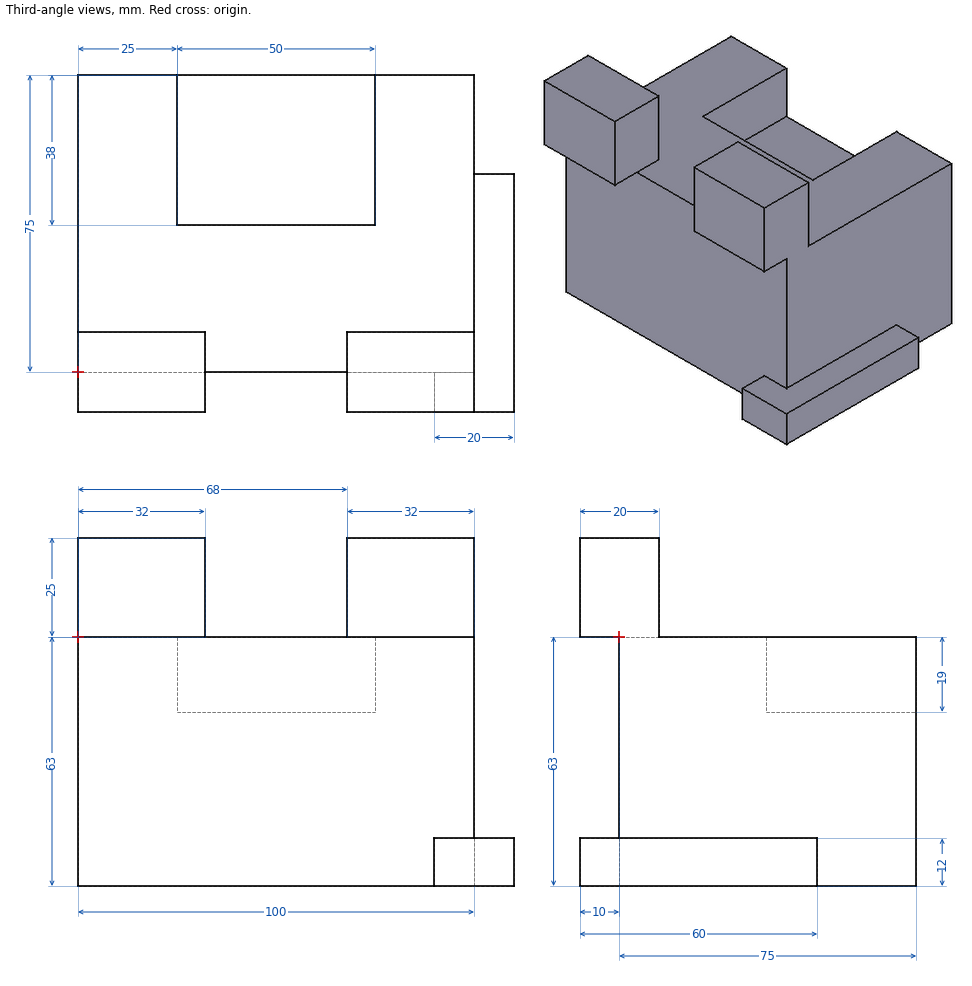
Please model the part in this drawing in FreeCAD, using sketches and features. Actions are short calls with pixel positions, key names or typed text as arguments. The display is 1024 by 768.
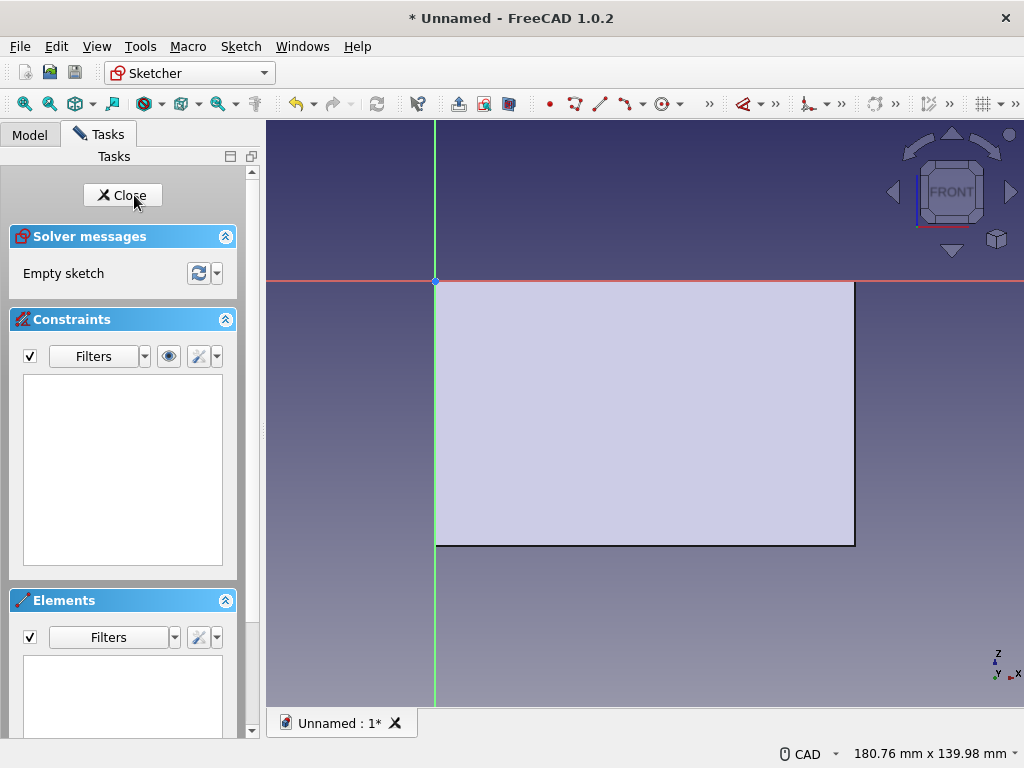
scroll(294, 679, down, 1)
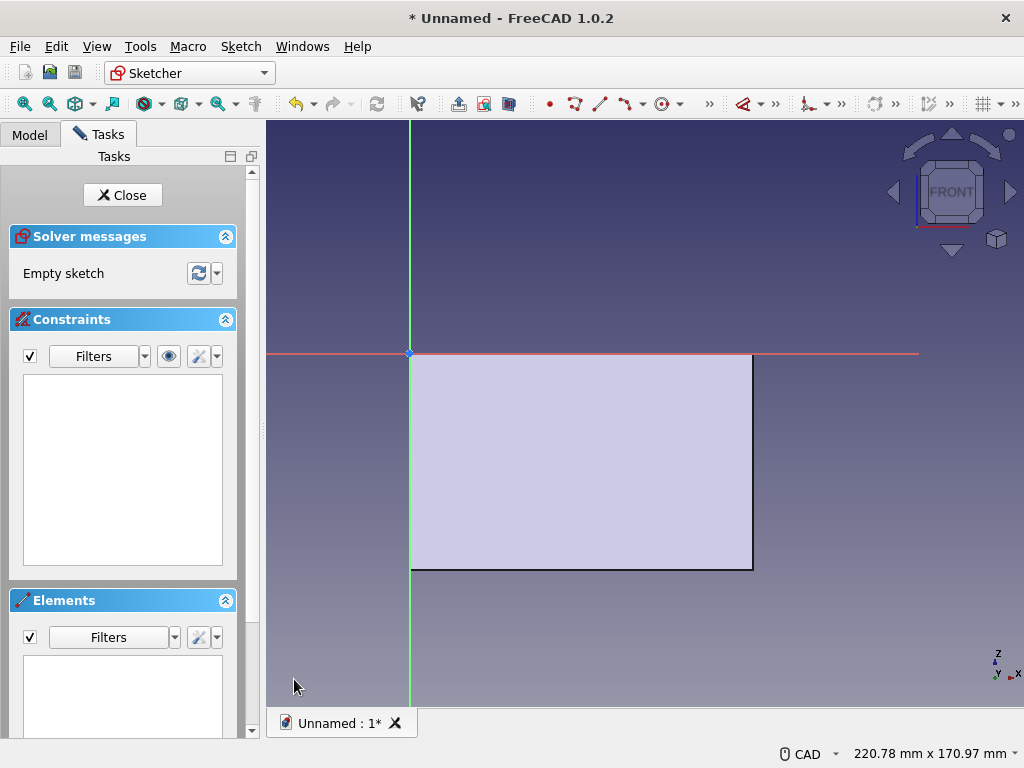
key(g)
key(r)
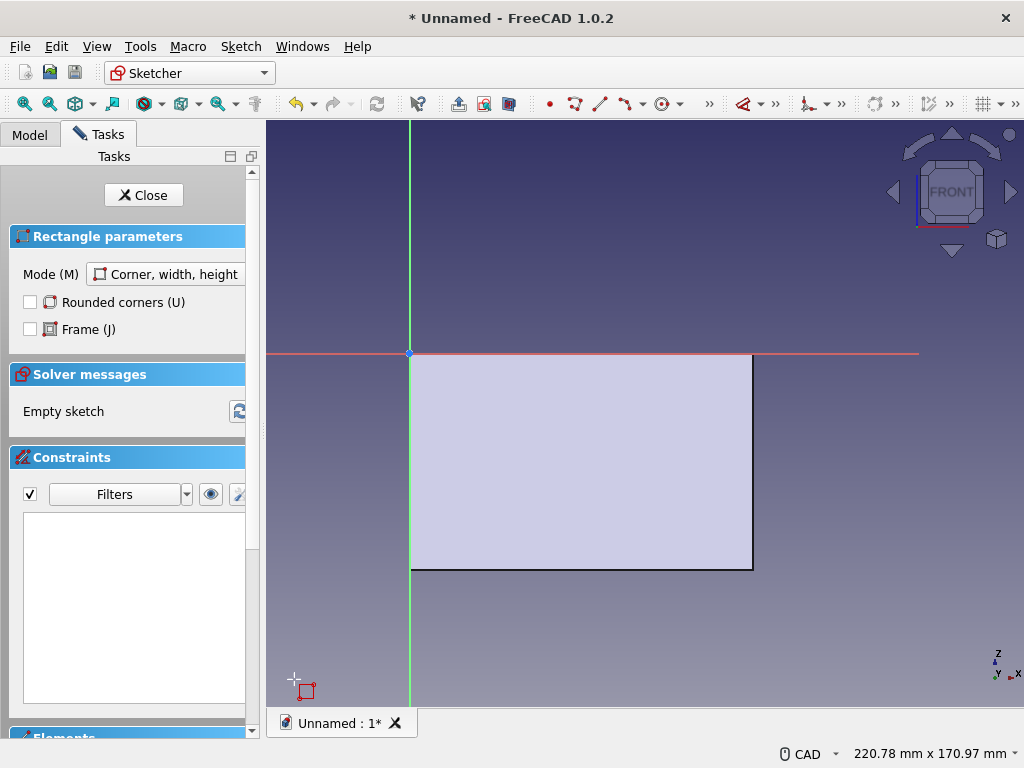
click(410, 354)
click(520, 268)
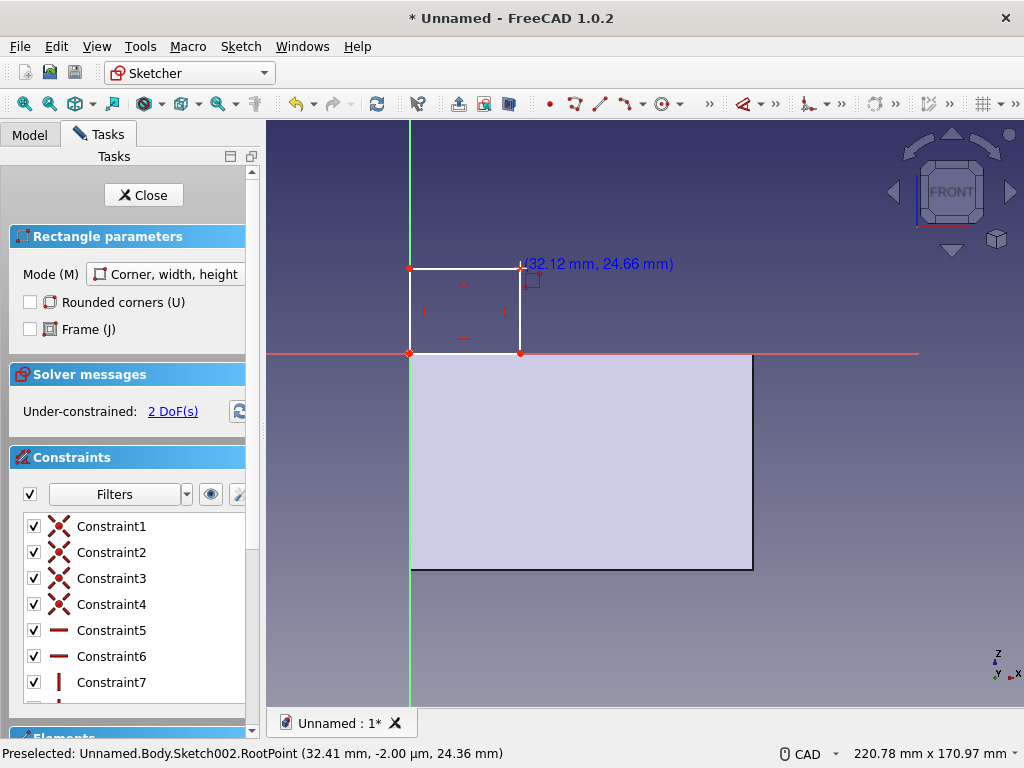
click(643, 268)
click(753, 354)
key(Escape)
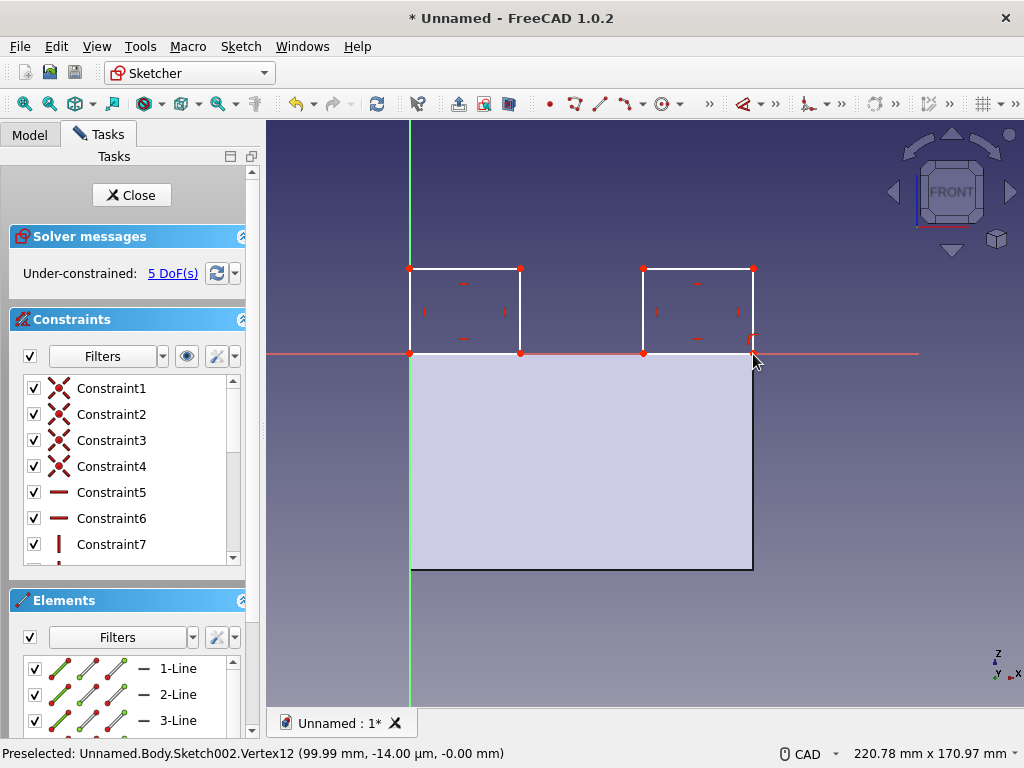
click(742, 104)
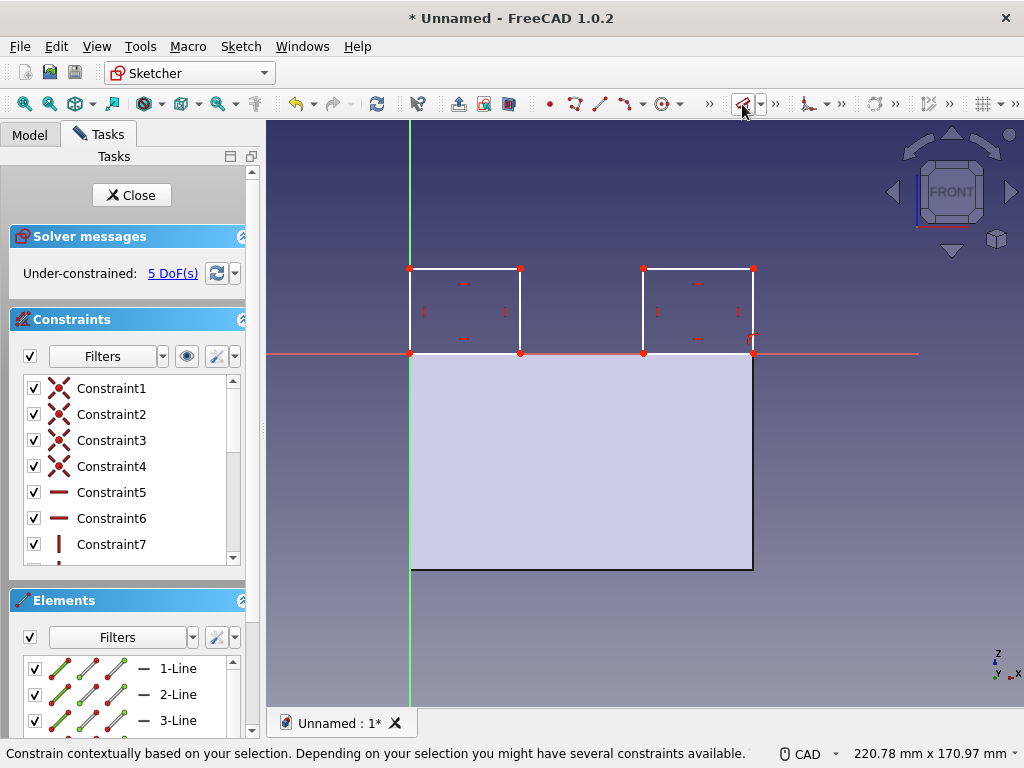
click(443, 354)
click(465, 388)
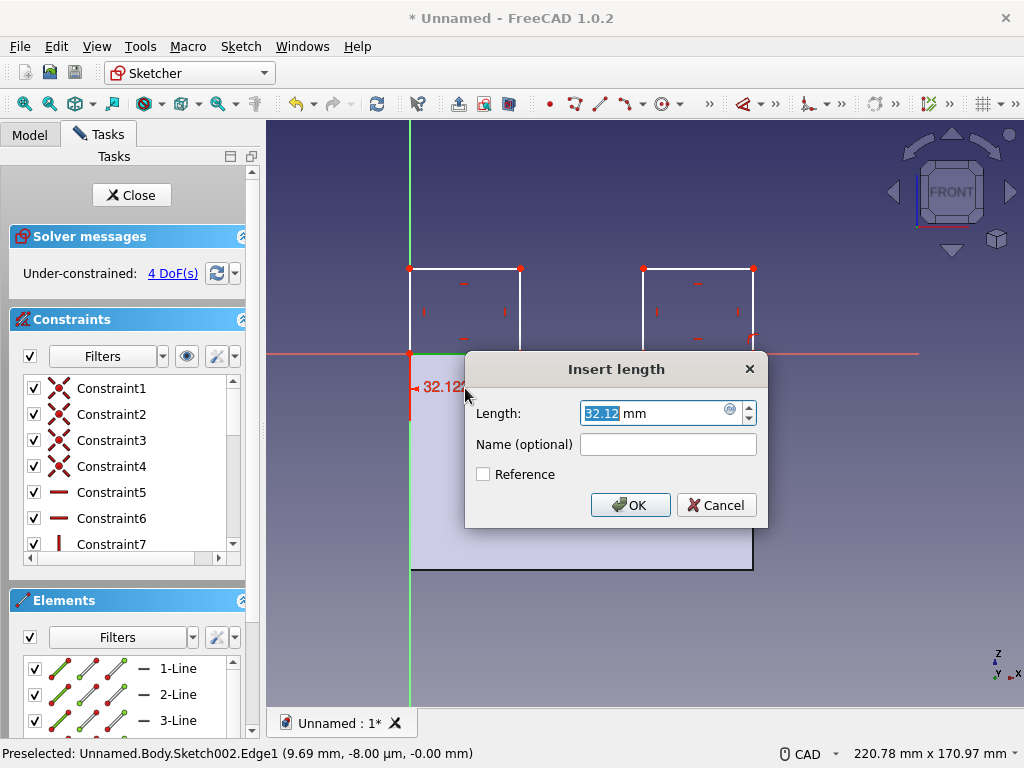
text(32)
key(Return)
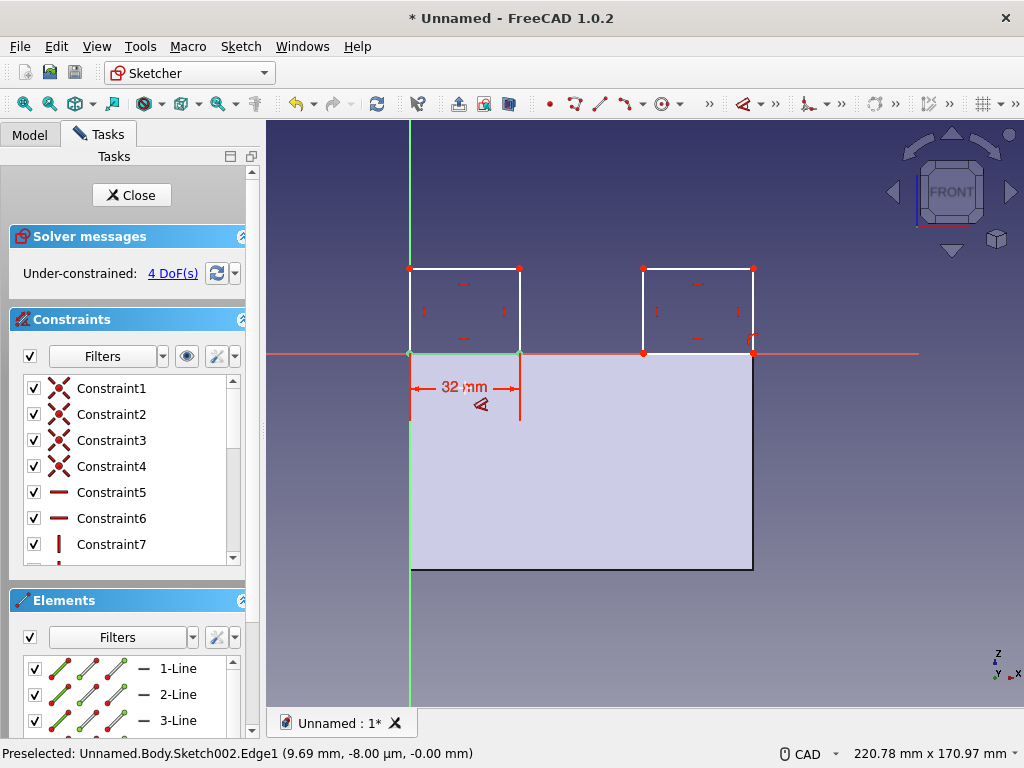
click(520, 328)
click(486, 311)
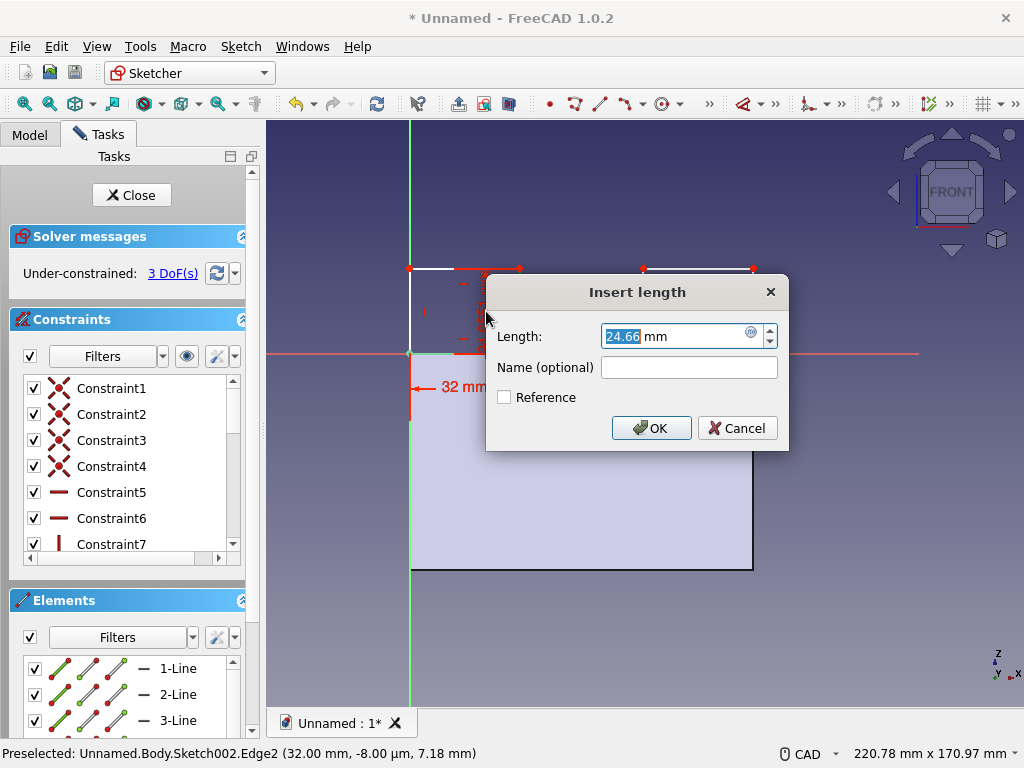
text(25)
key(Return)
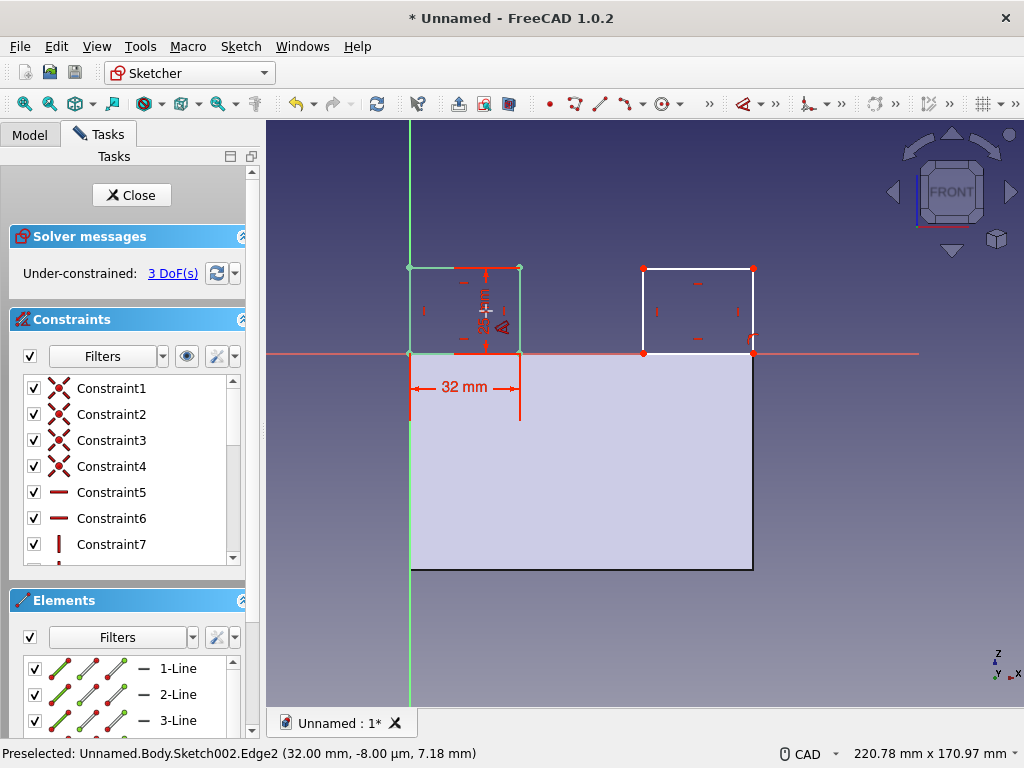
click(643, 294)
click(677, 311)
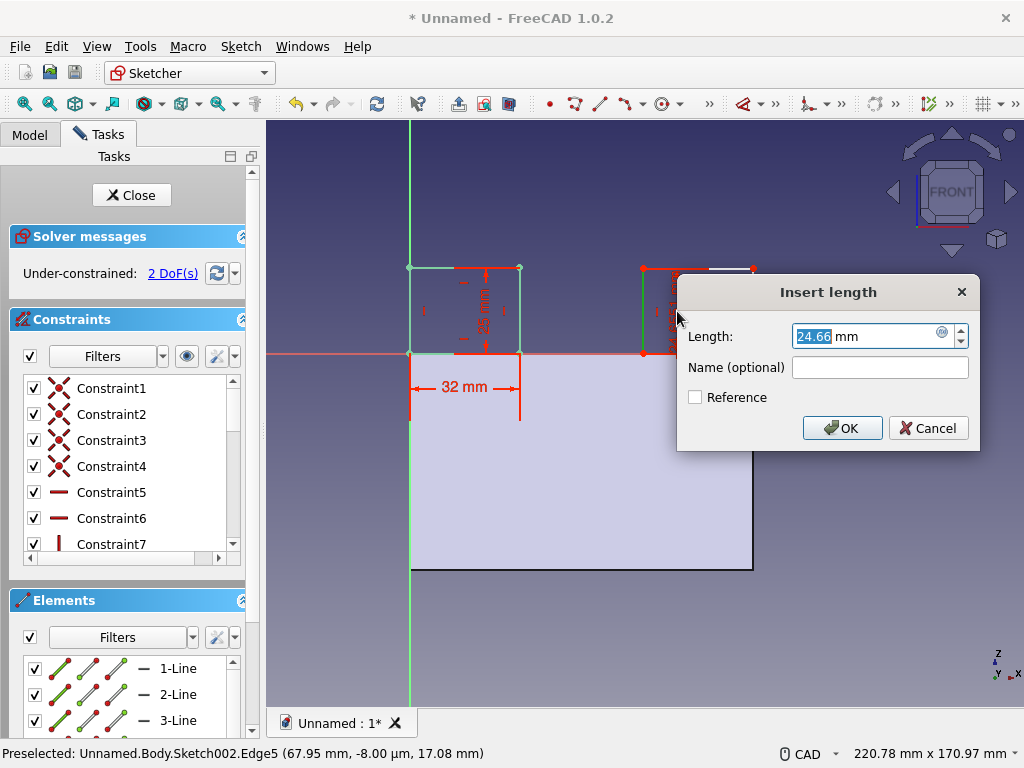
text(25)
key(Return)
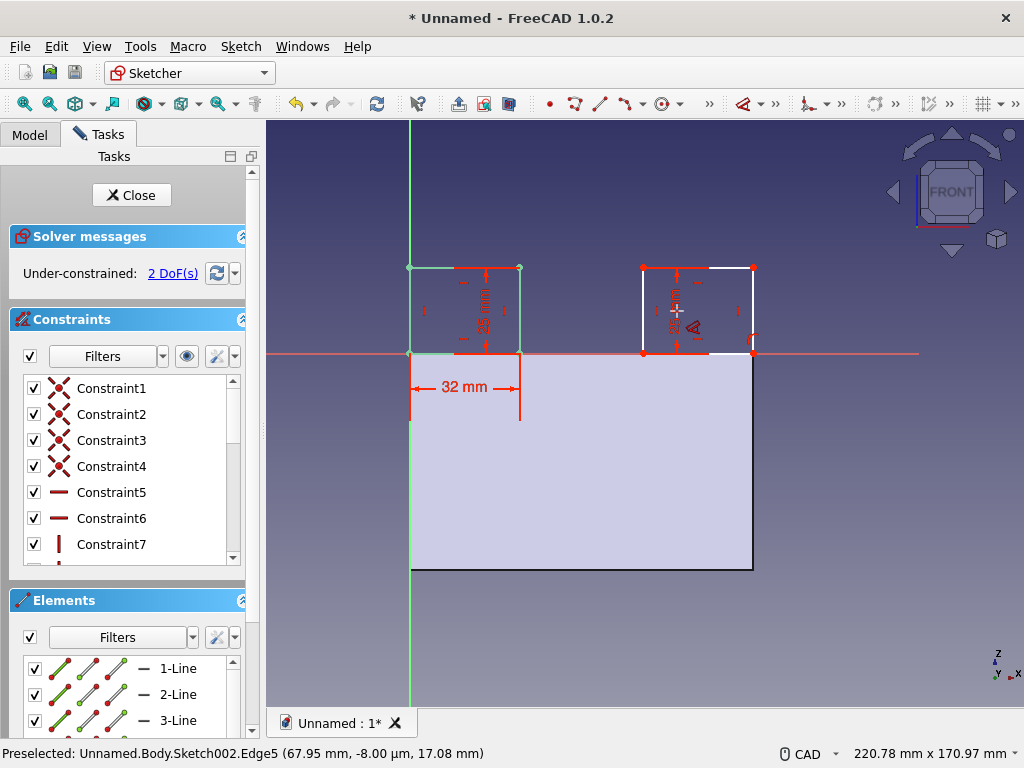
click(676, 354)
click(698, 388)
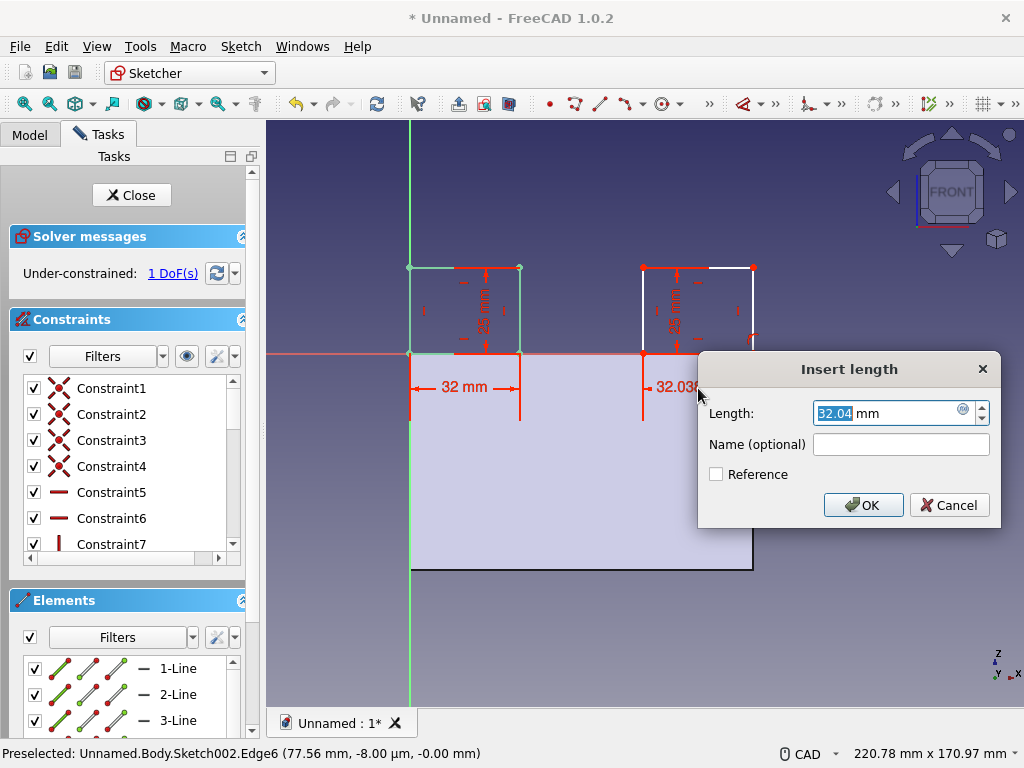
text(32)
key(Return)